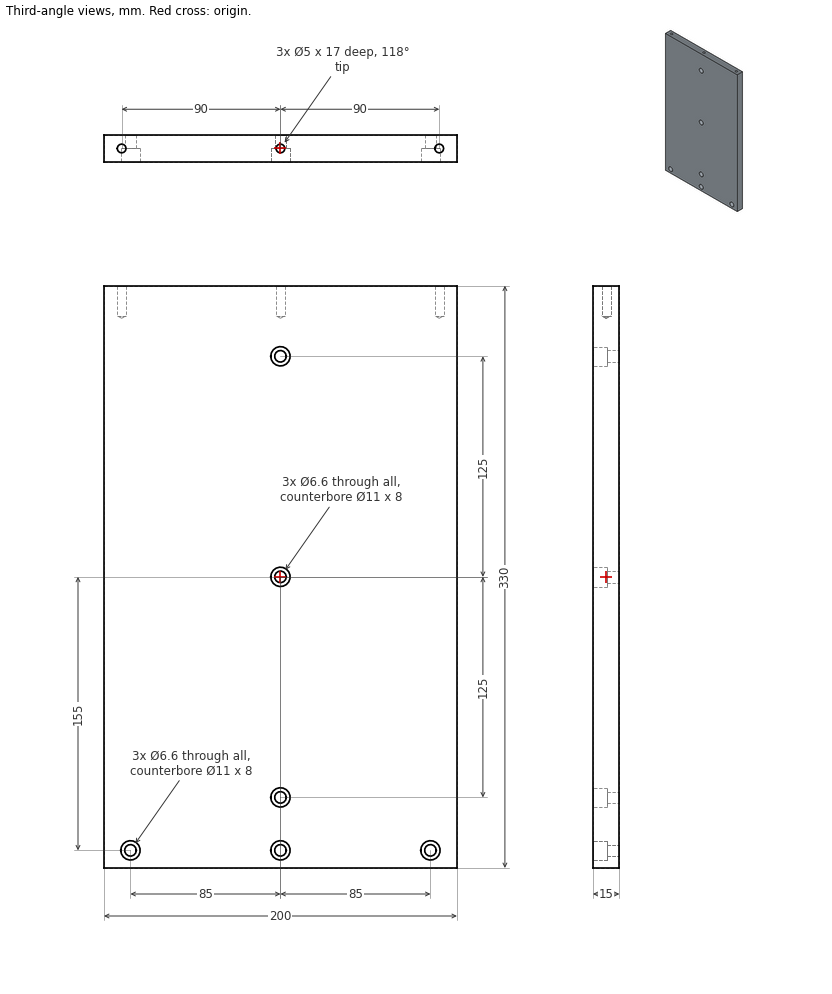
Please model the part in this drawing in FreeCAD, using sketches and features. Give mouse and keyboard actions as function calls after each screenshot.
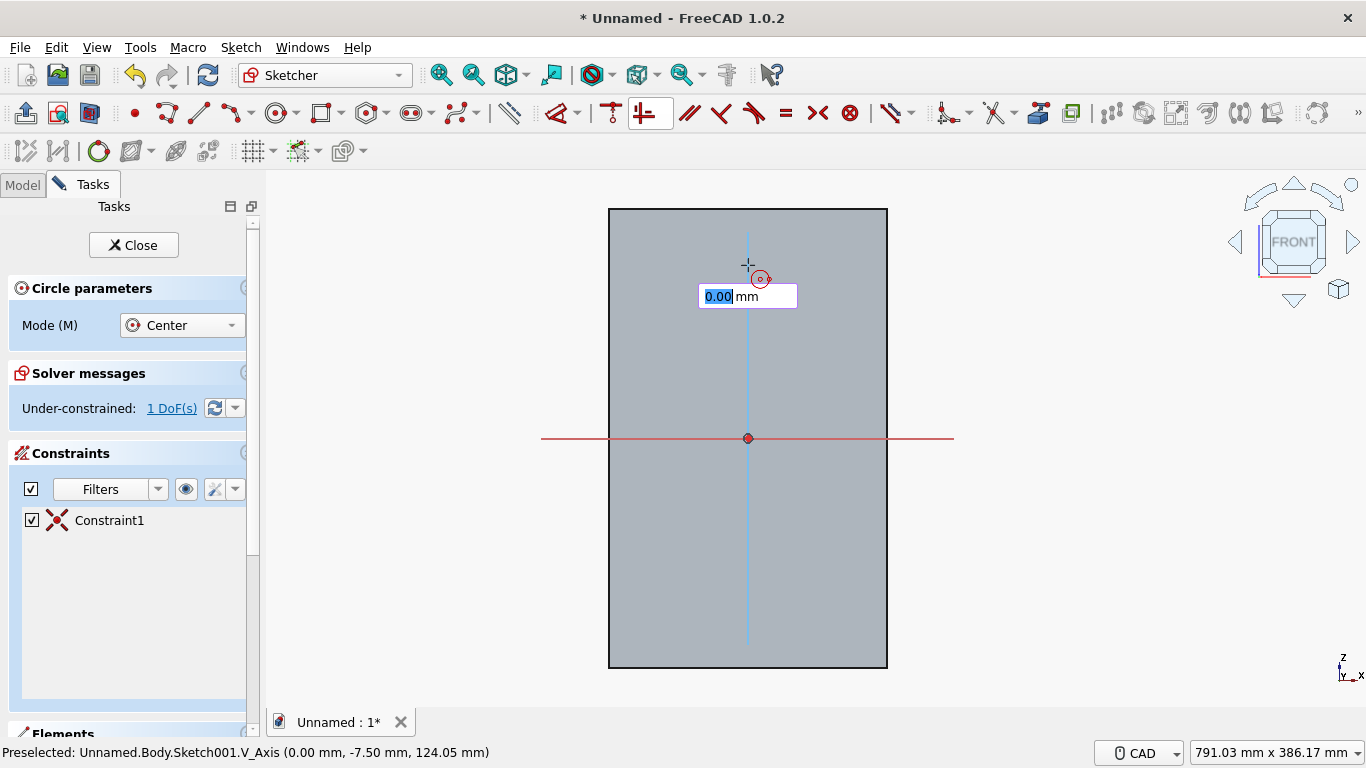
scroll(752, 263, up, 7)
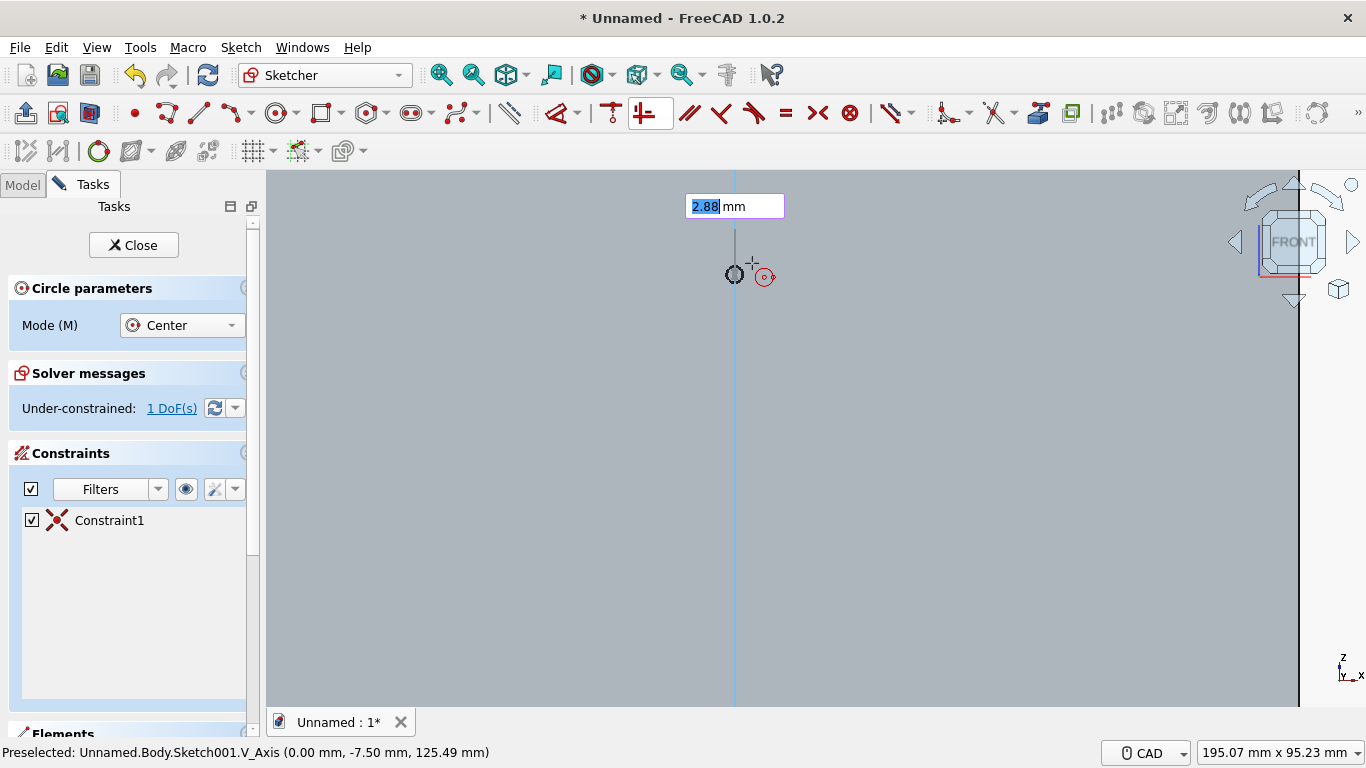
click(752, 263)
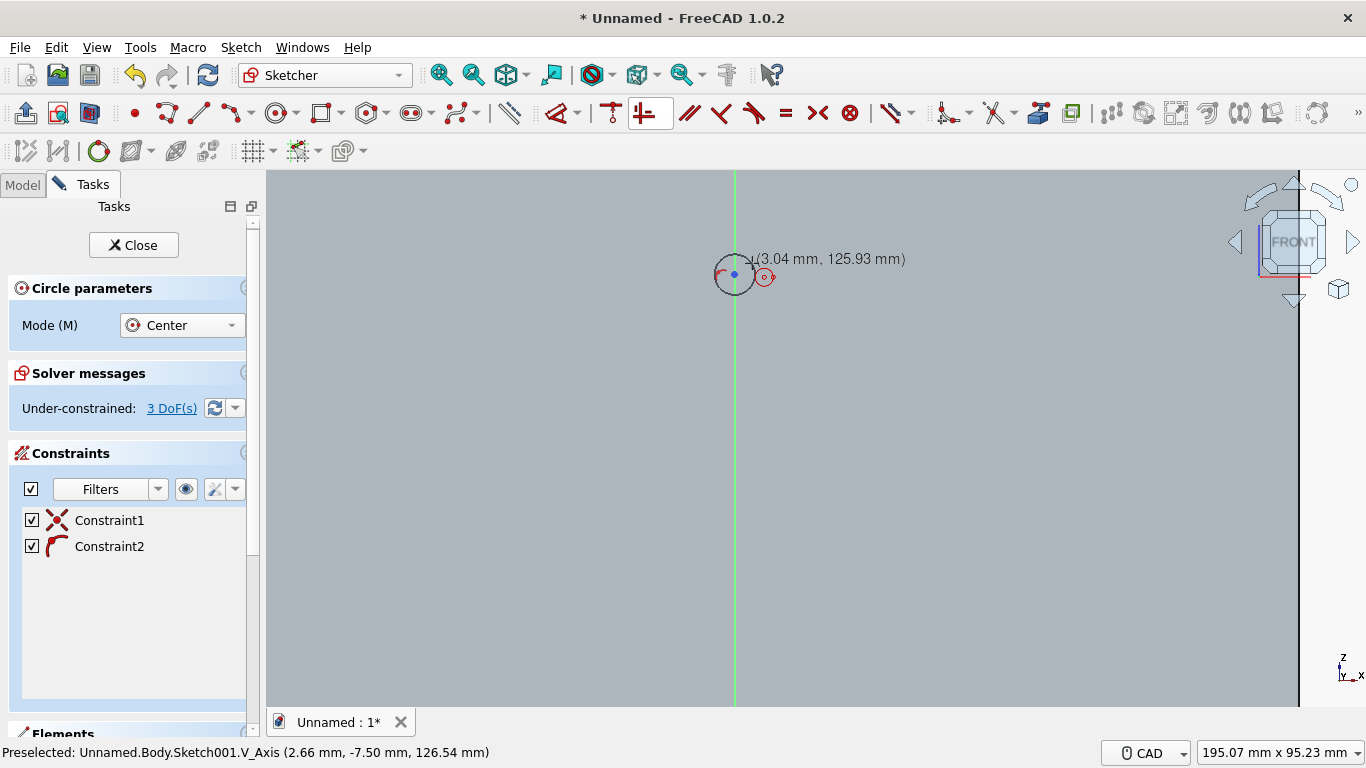
scroll(752, 263, down, 7)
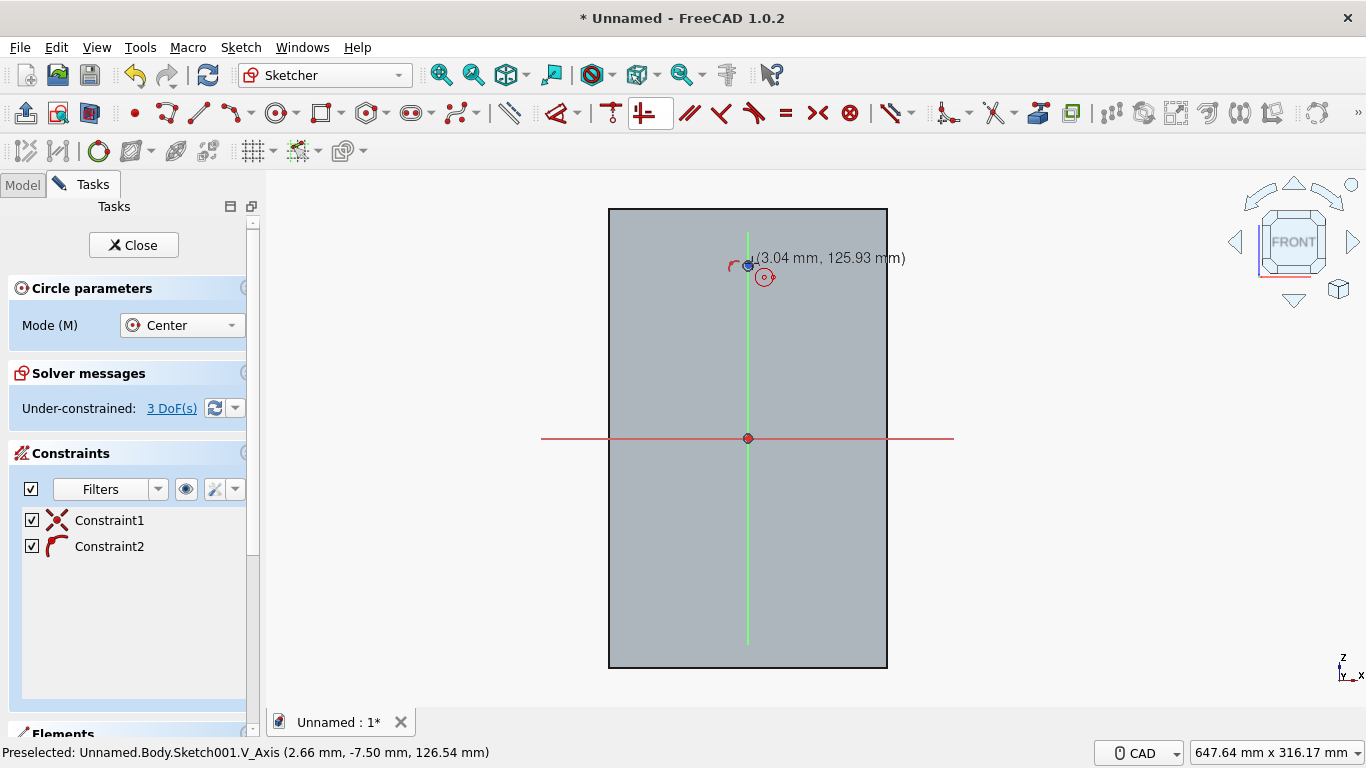
scroll(748, 612, up, 8)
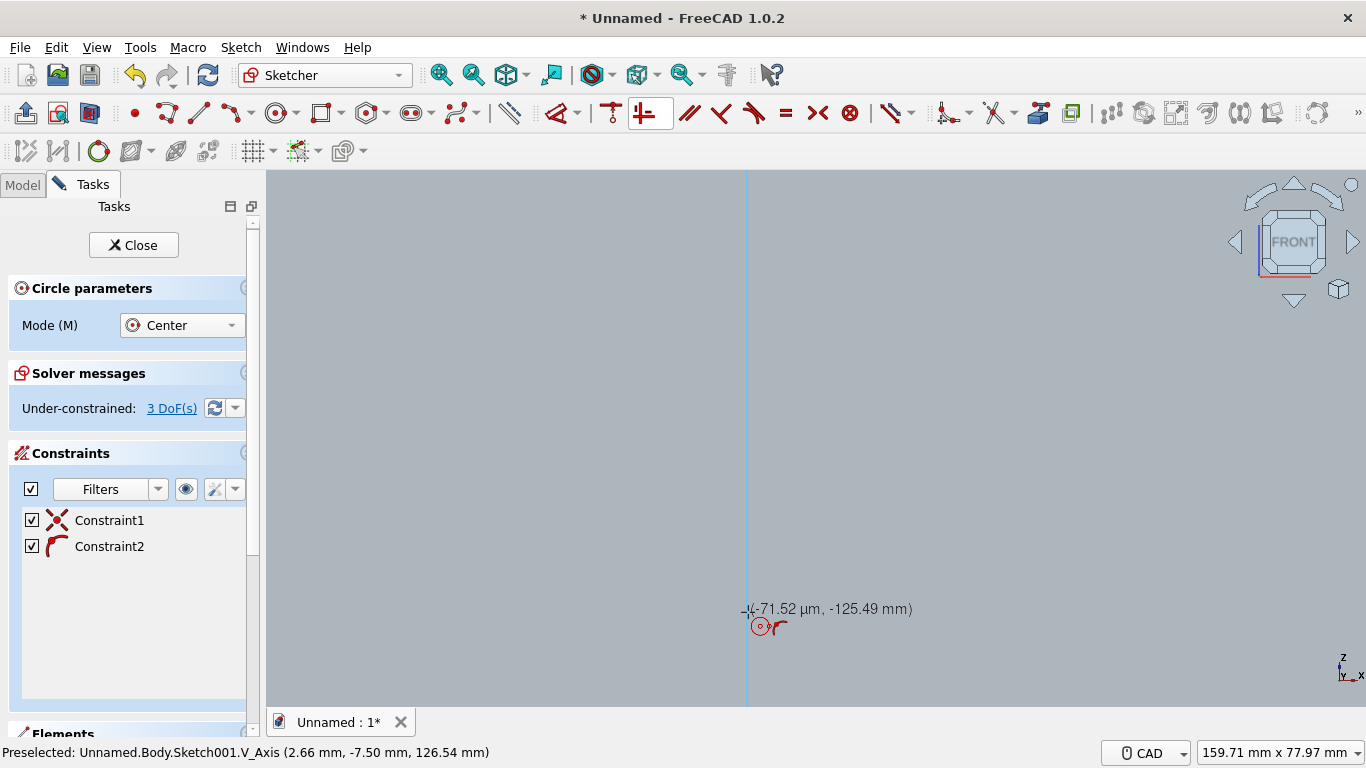
scroll(748, 613, down, 8)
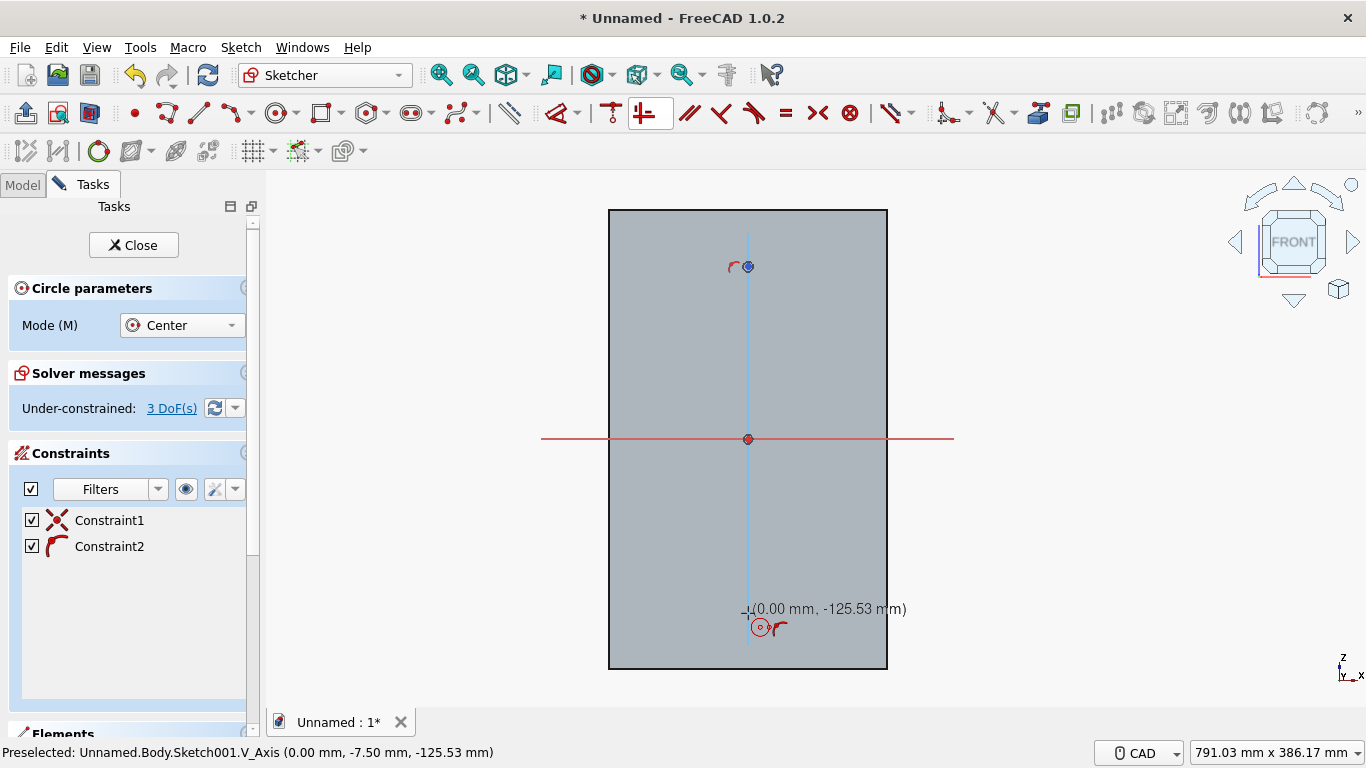
click(748, 613)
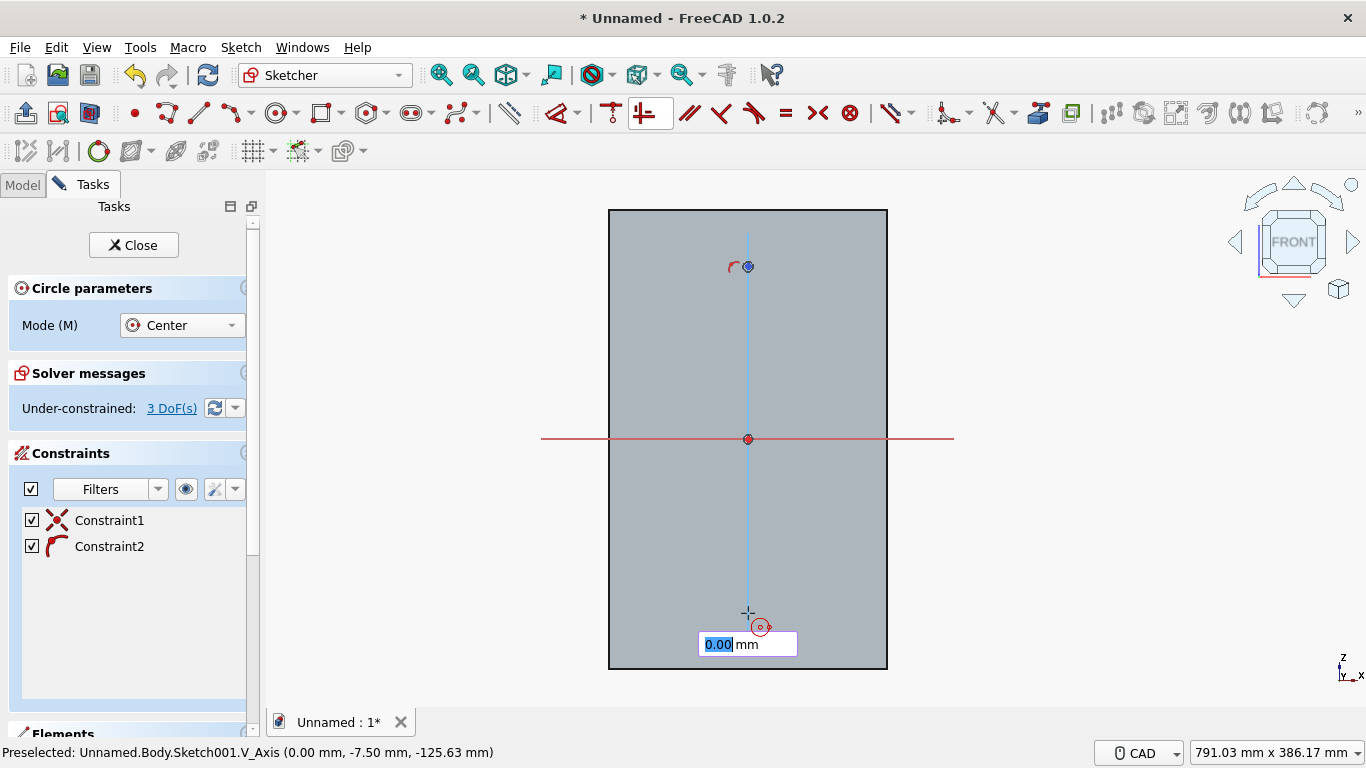
scroll(752, 612, up, 7)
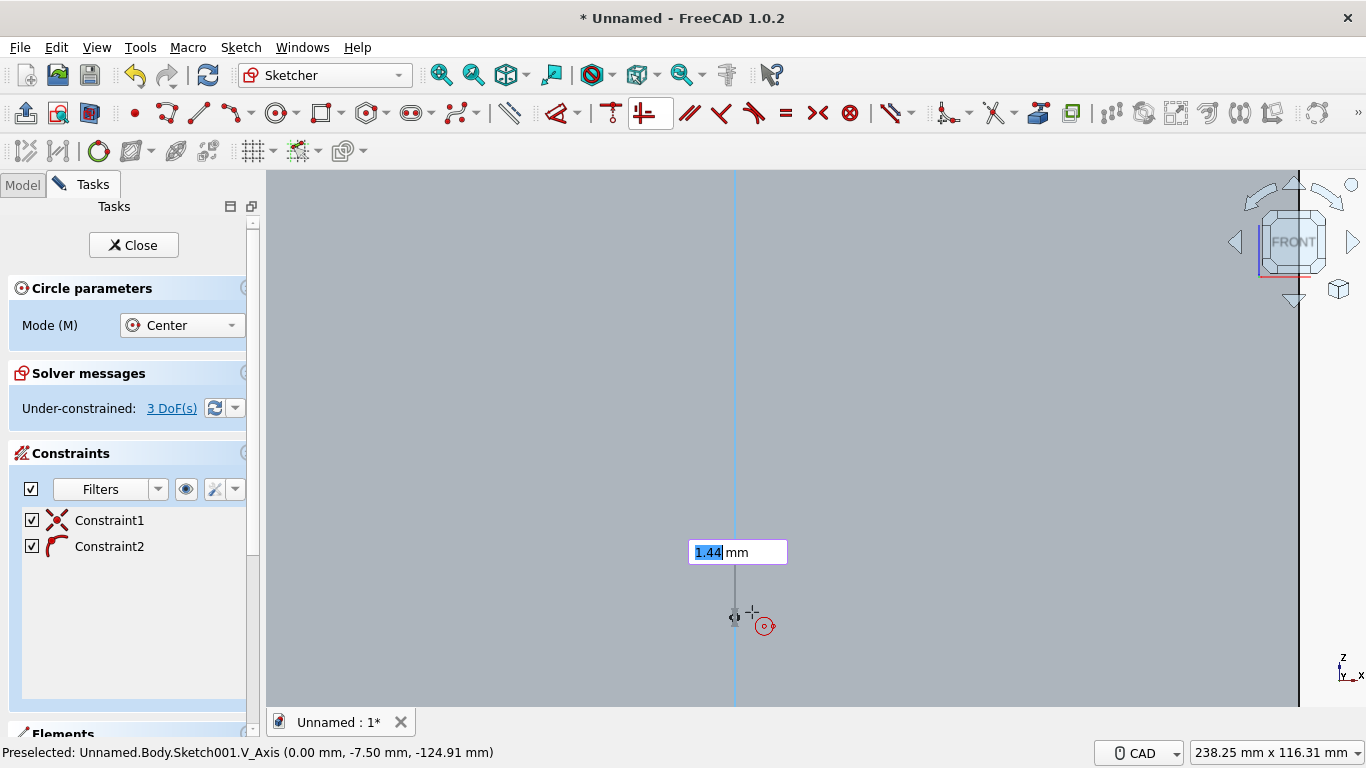
click(752, 608)
key(Escape)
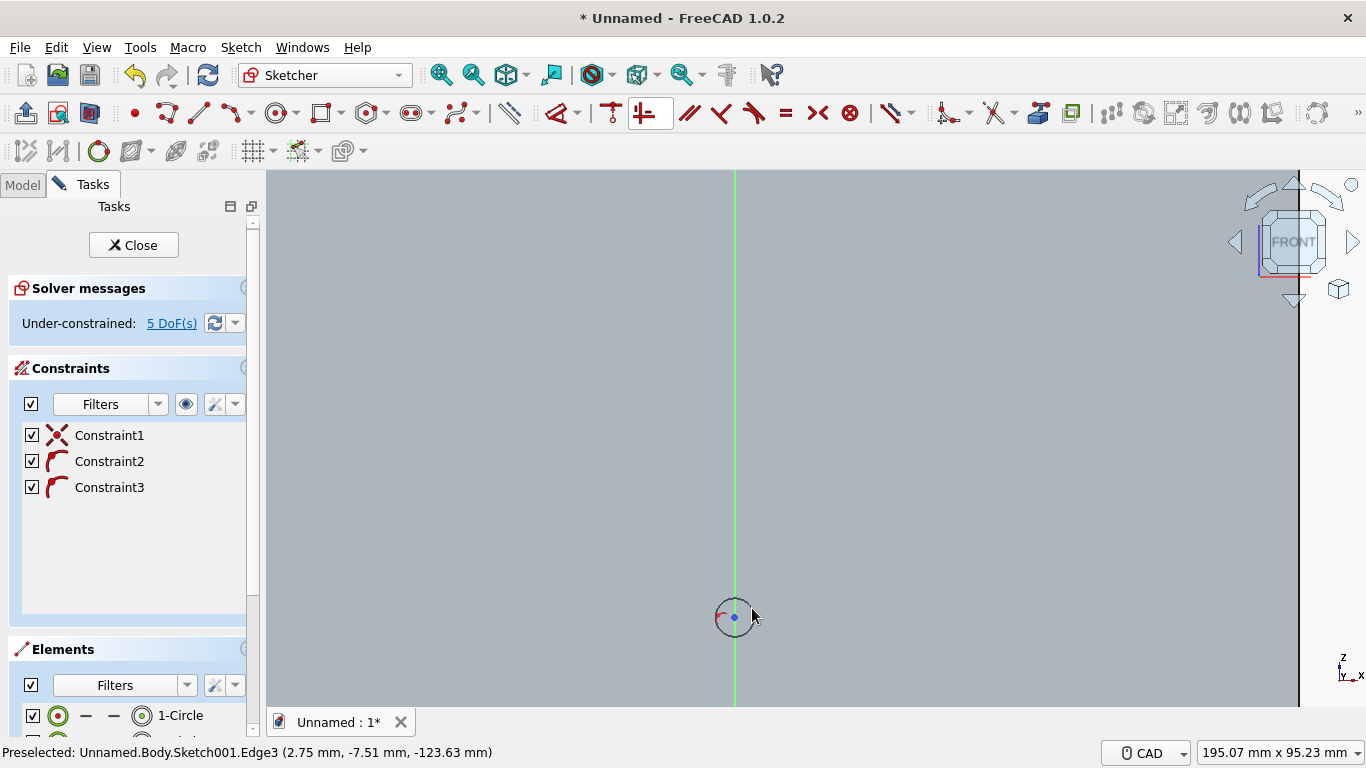
scroll(752, 612, down, 7)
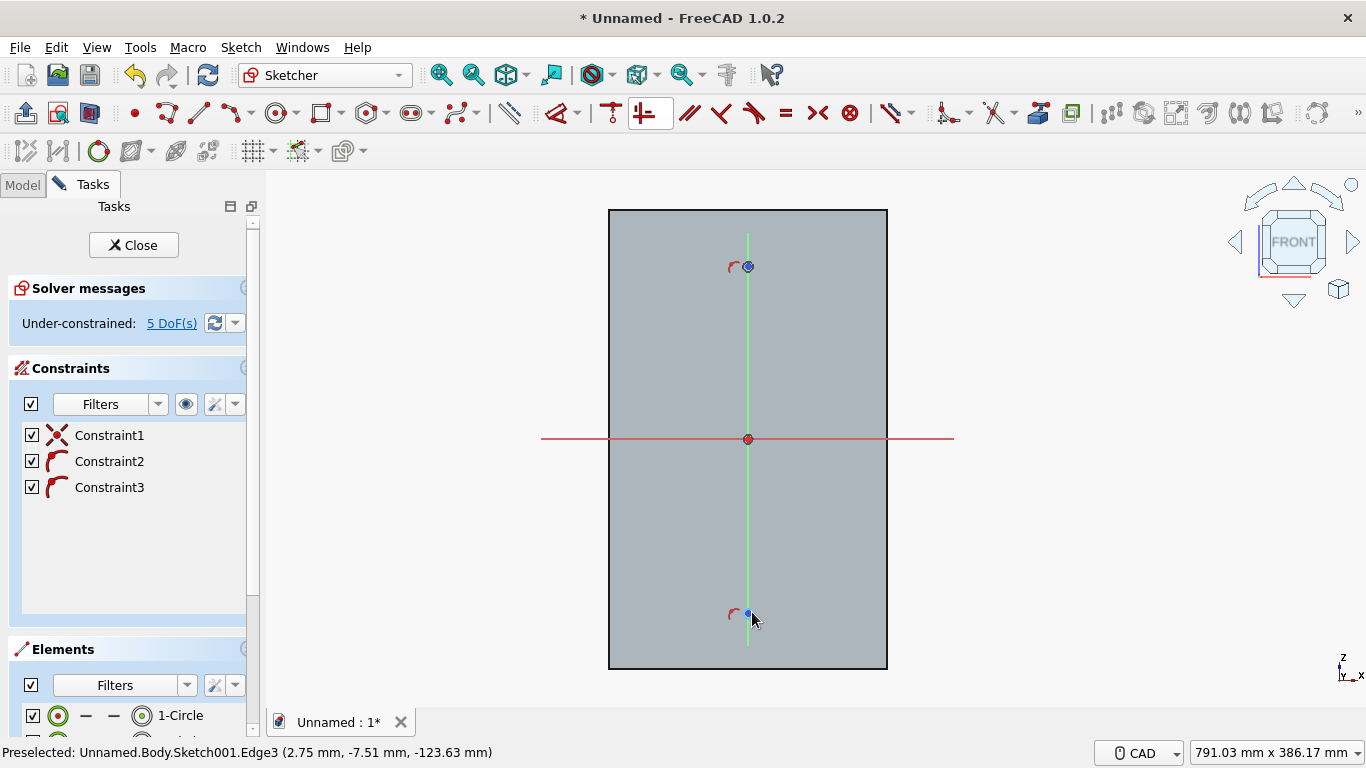
scroll(751, 436, up, 8)